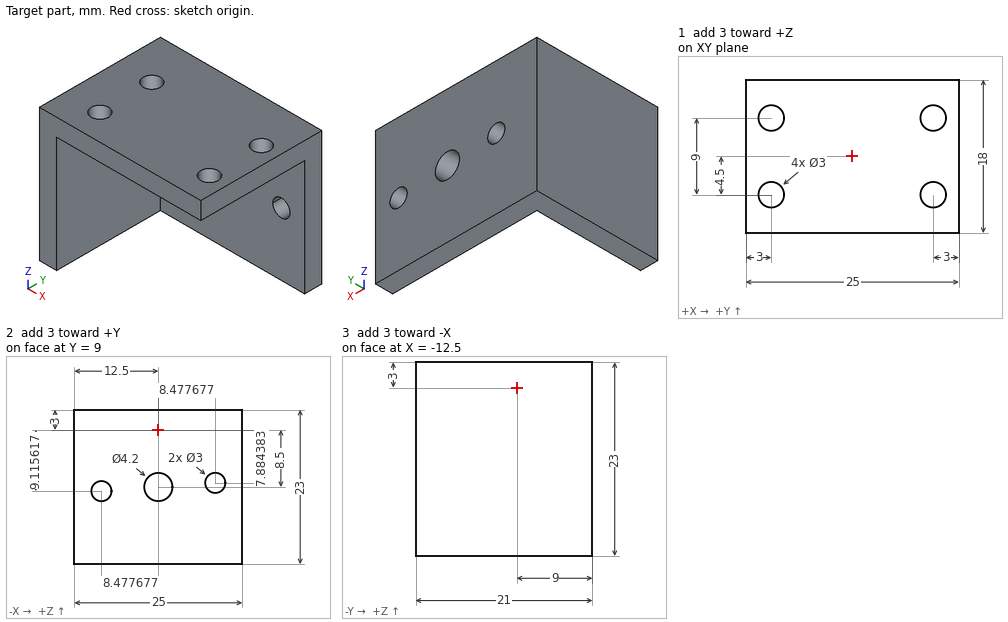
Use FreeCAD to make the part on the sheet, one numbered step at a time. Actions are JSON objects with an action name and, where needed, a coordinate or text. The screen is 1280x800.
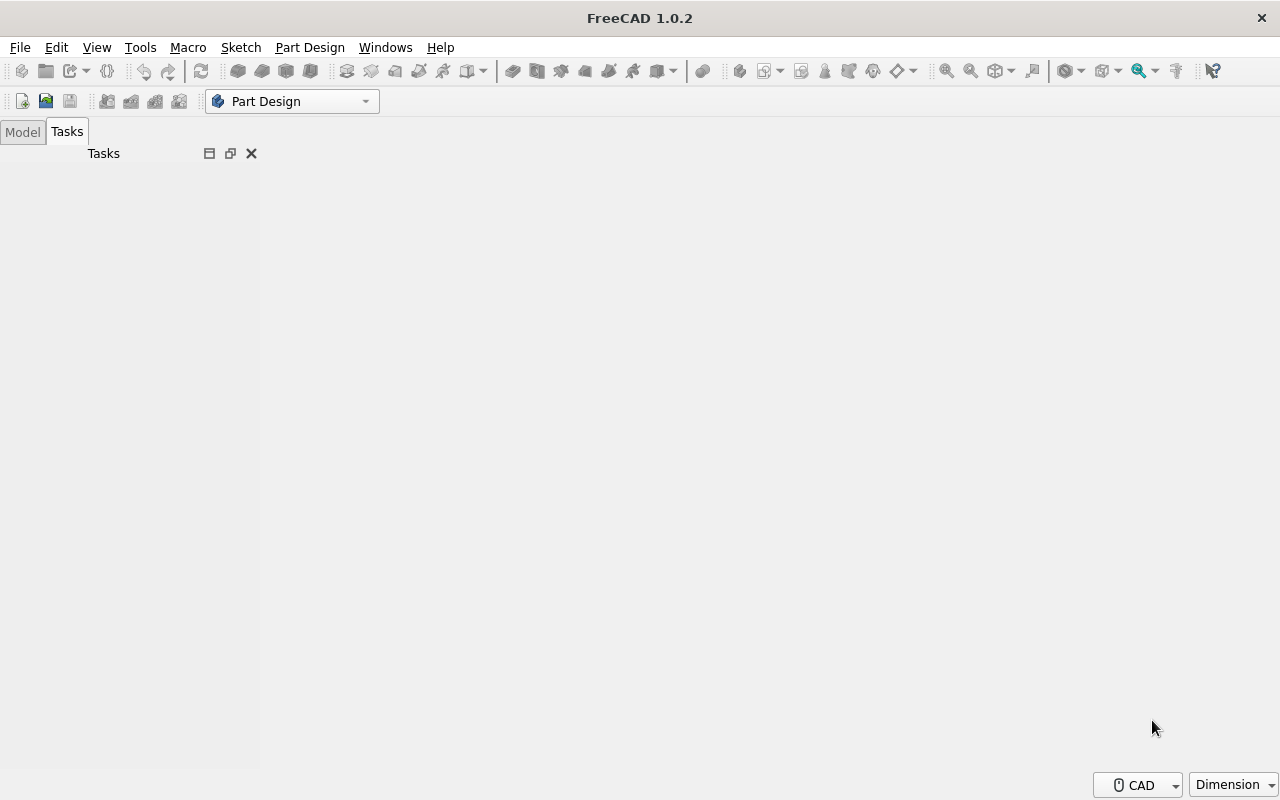
{"action": "key", "text": "ctrl+n"}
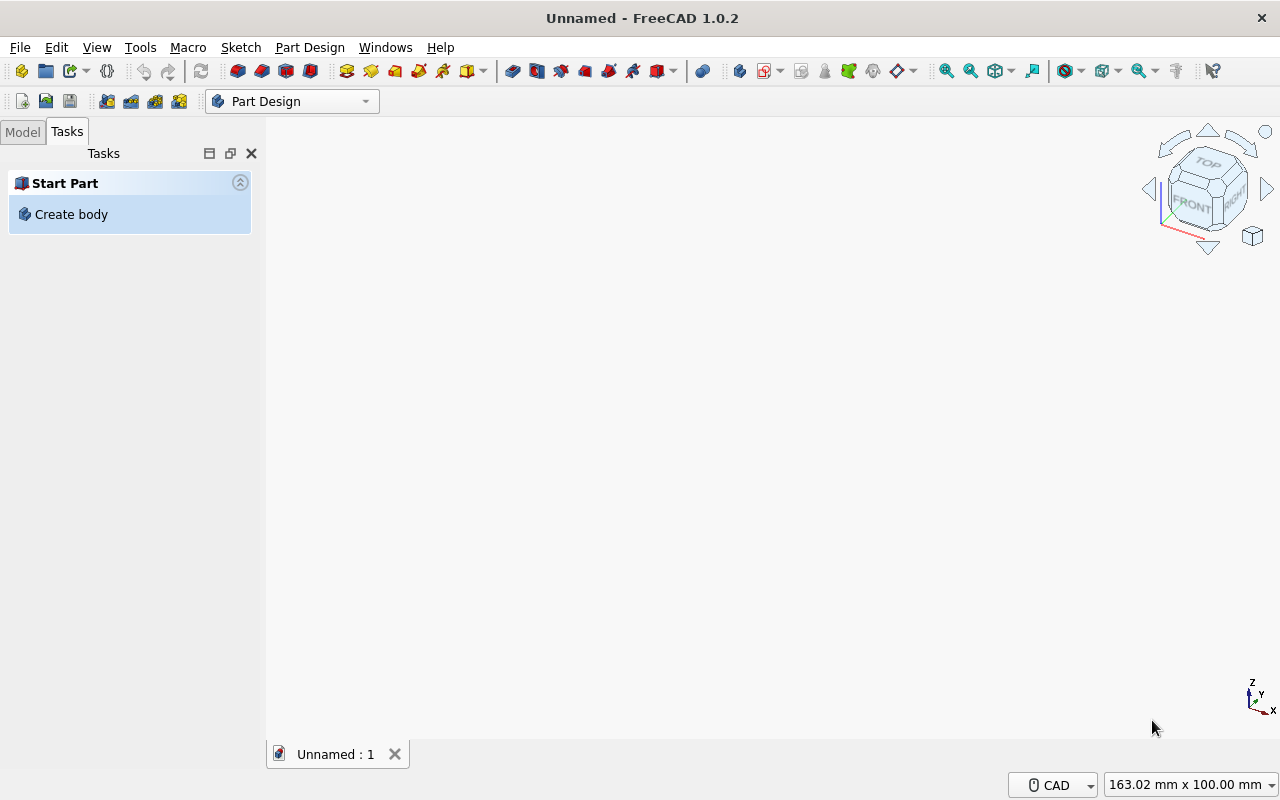
{"action": "left_click", "coordinate": [764, 72]}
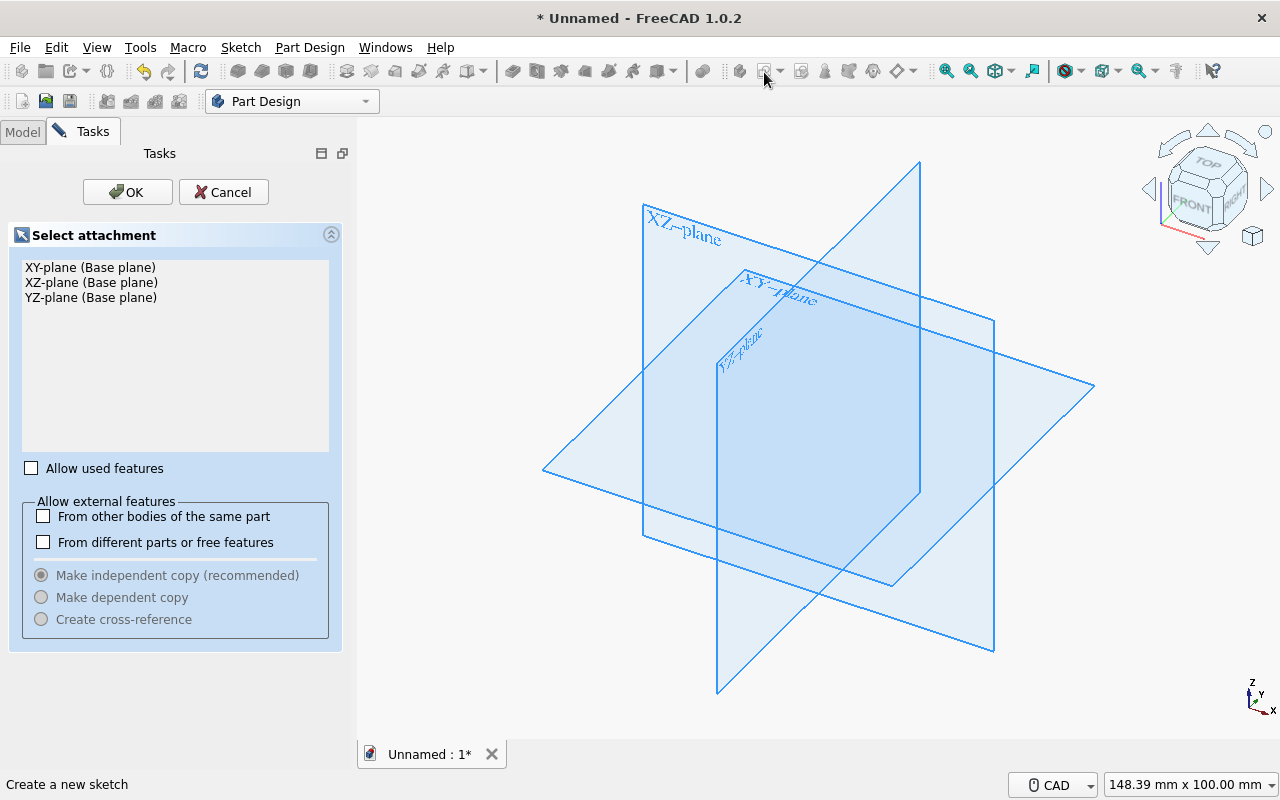
{"action": "left_click", "coordinate": [82, 268]}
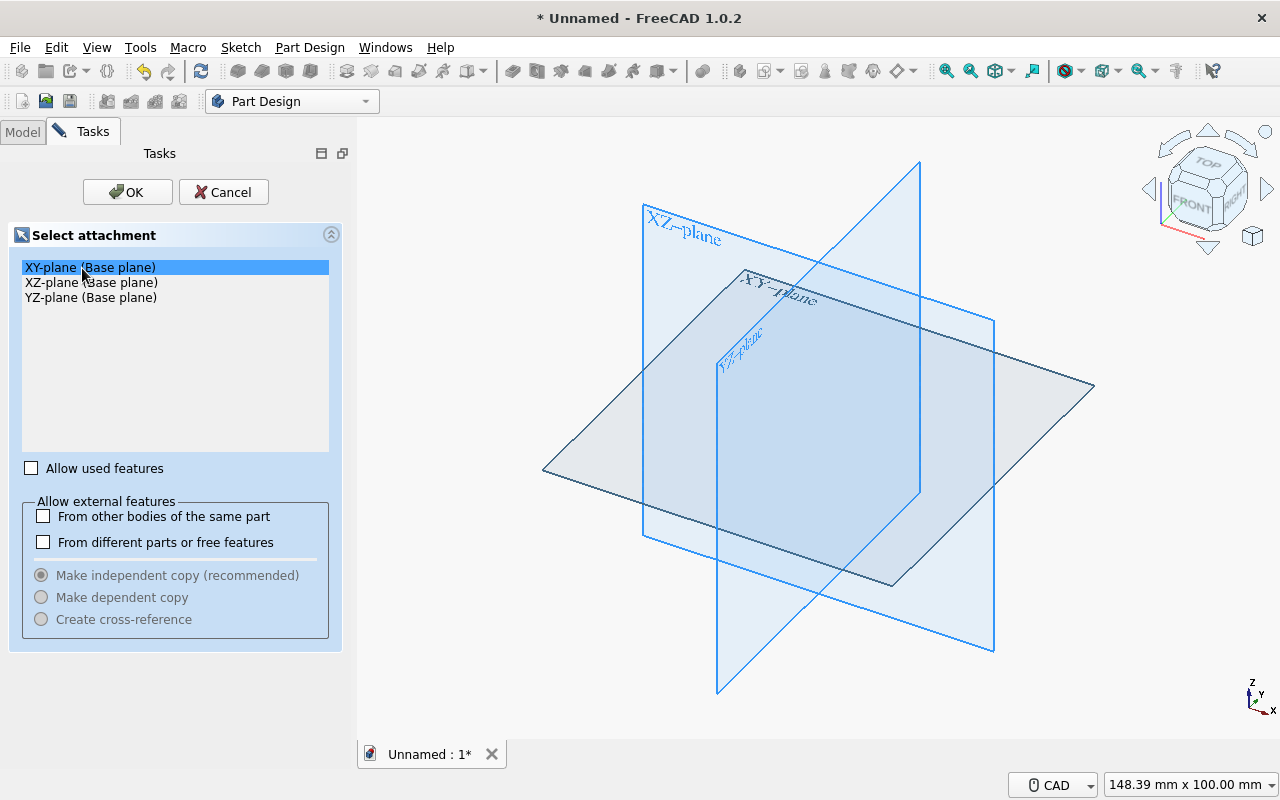
{"action": "left_click", "coordinate": [128, 192]}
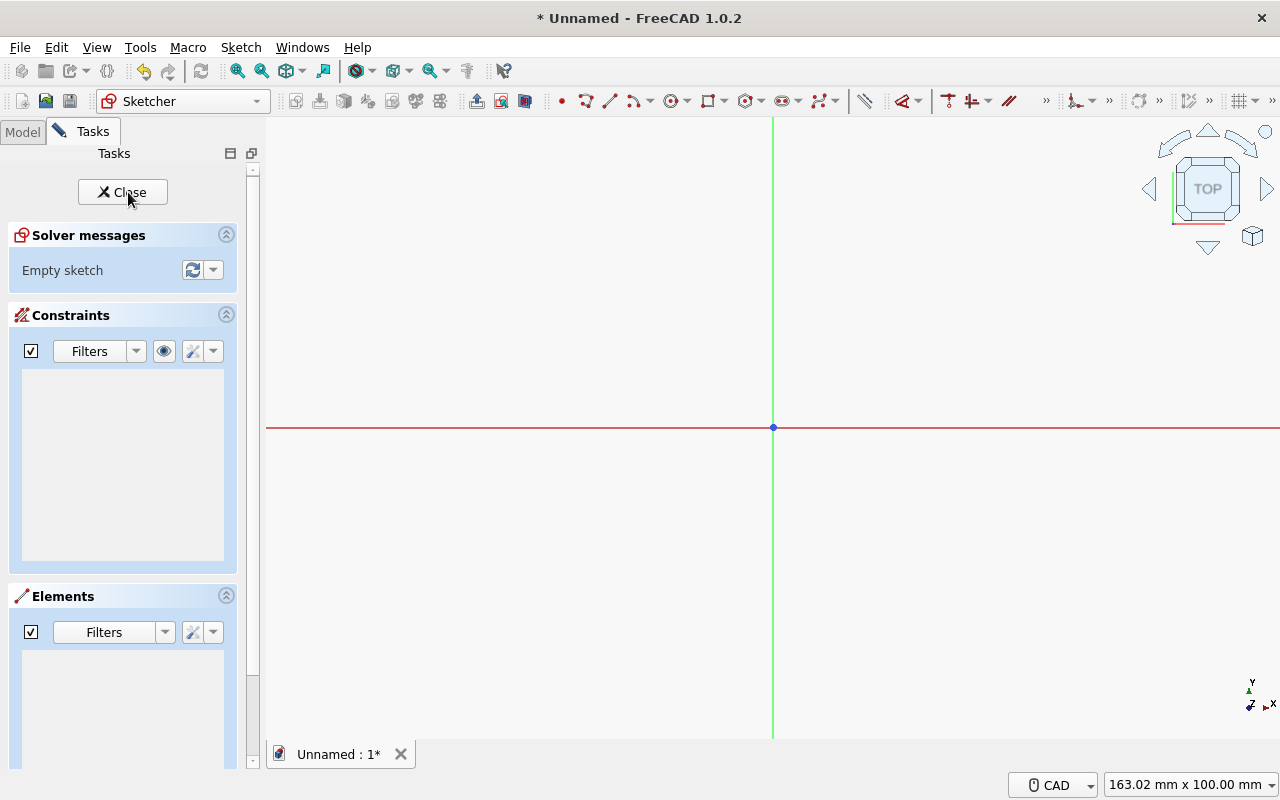
{"action": "scroll", "coordinate": [803, 428], "scroll_direction": "up", "scroll_amount": 6}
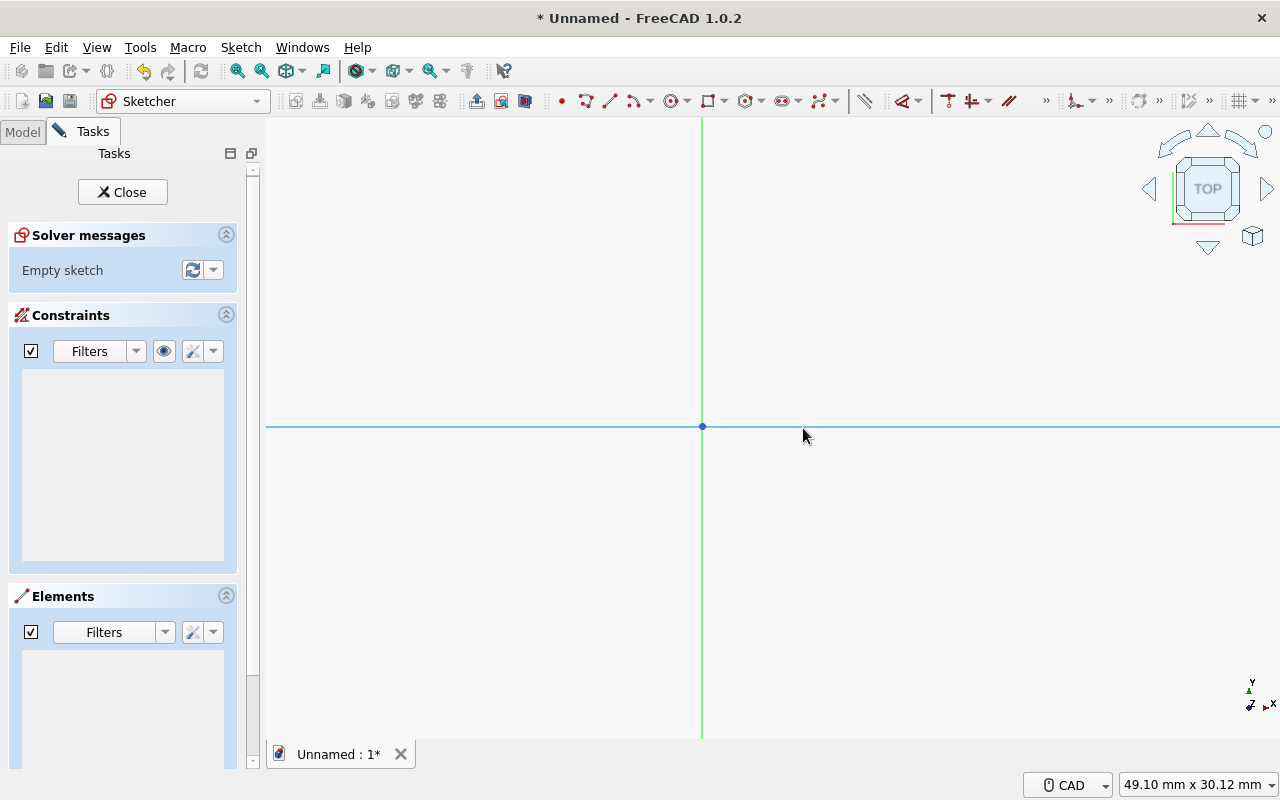
{"action": "key", "text": "g v"}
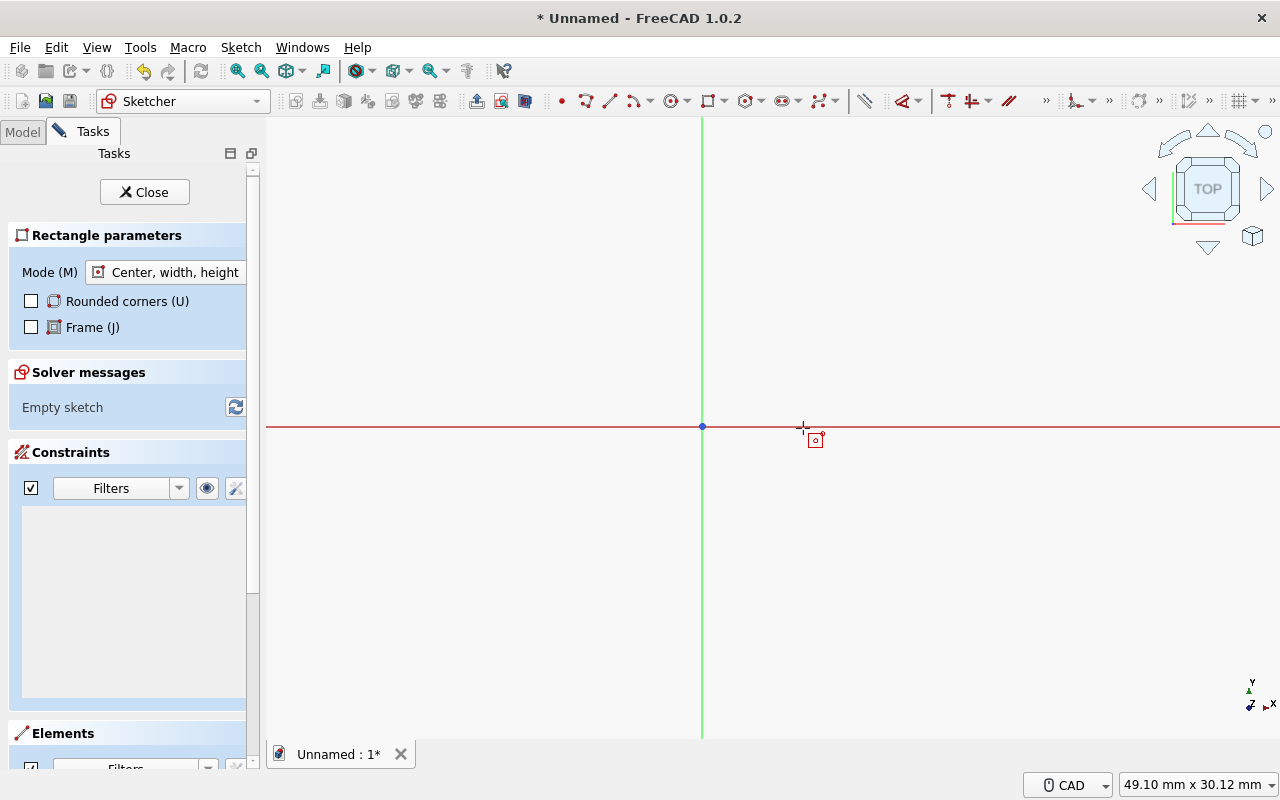
{"action": "left_click", "coordinate": [702, 427]}
{"action": "mouse_move", "coordinate": [960, 241]}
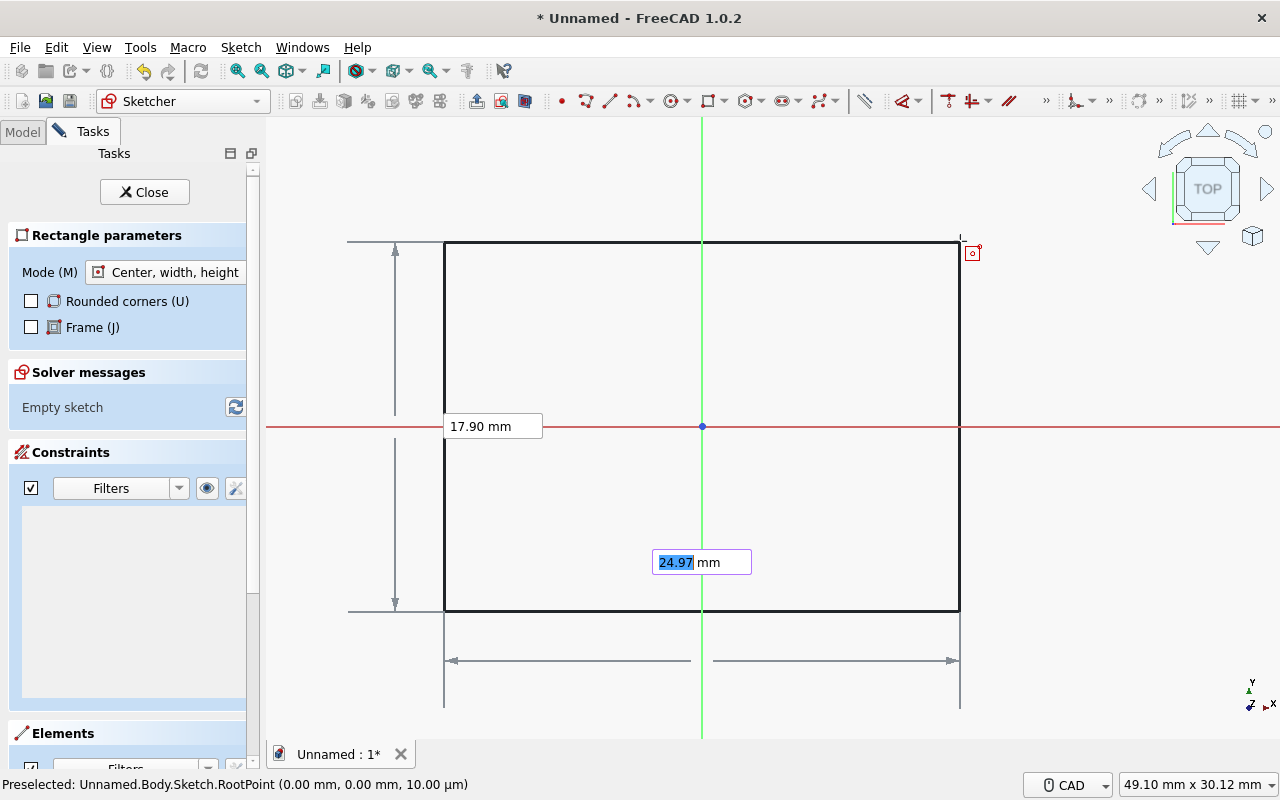
{"action": "type", "text": "25"}
{"action": "key", "text": "Tab"}
{"action": "type", "text": "18"}
{"action": "key", "text": "Return"}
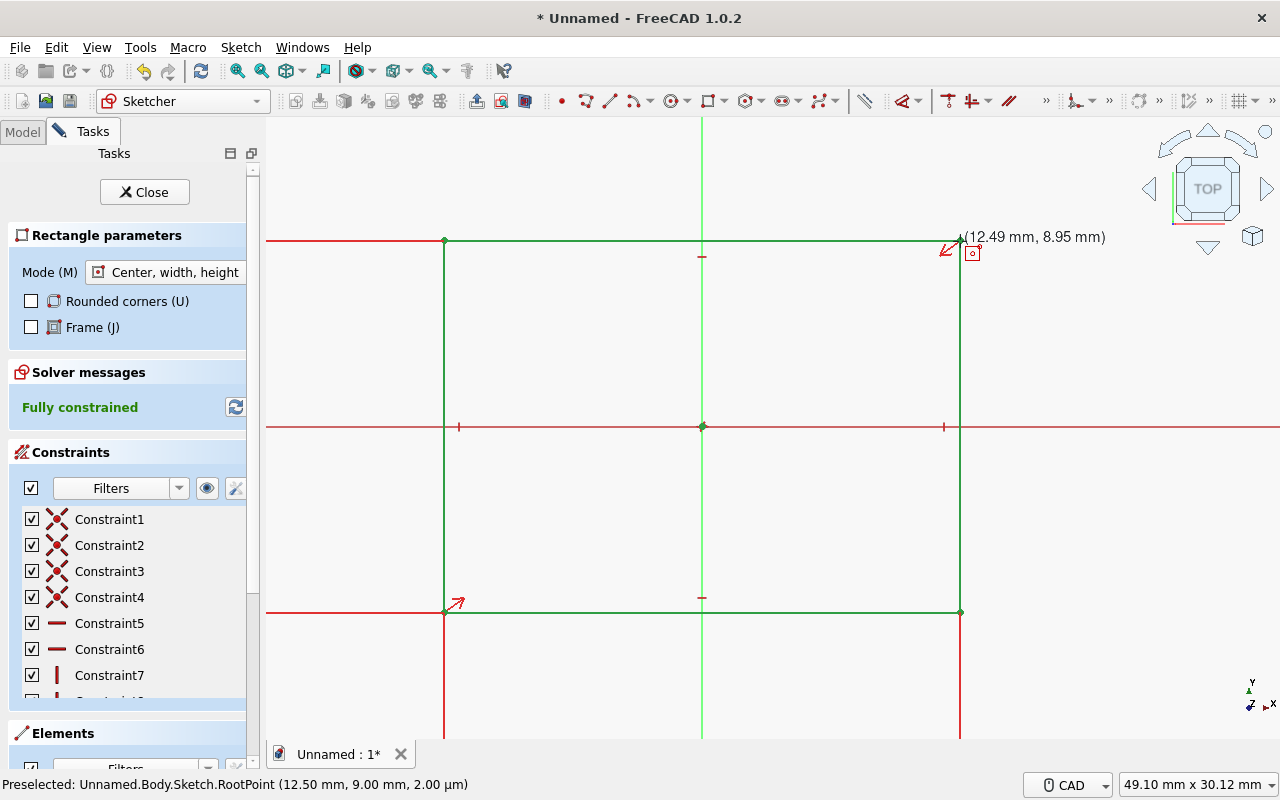
{"action": "key", "text": "g c"}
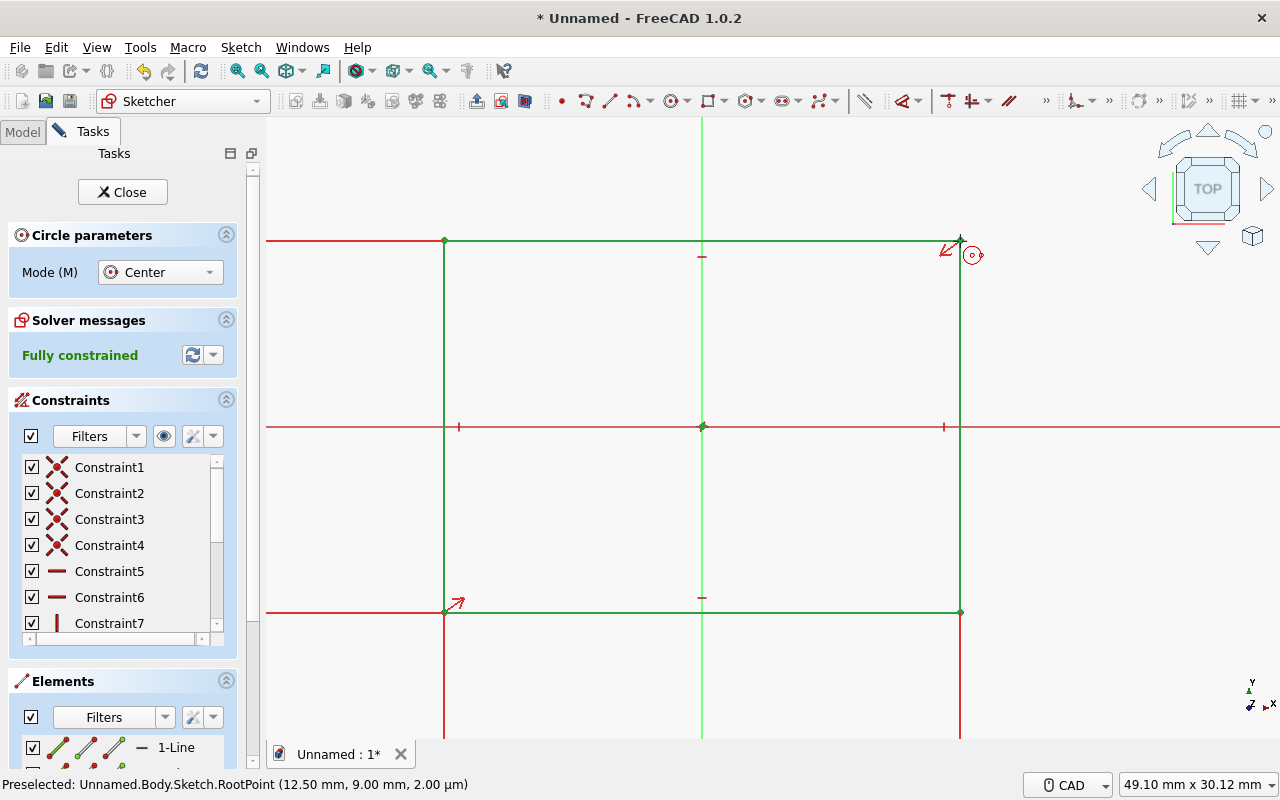
{"action": "left_click", "coordinate": [506, 520]}
{"action": "mouse_move", "coordinate": [528, 498]}